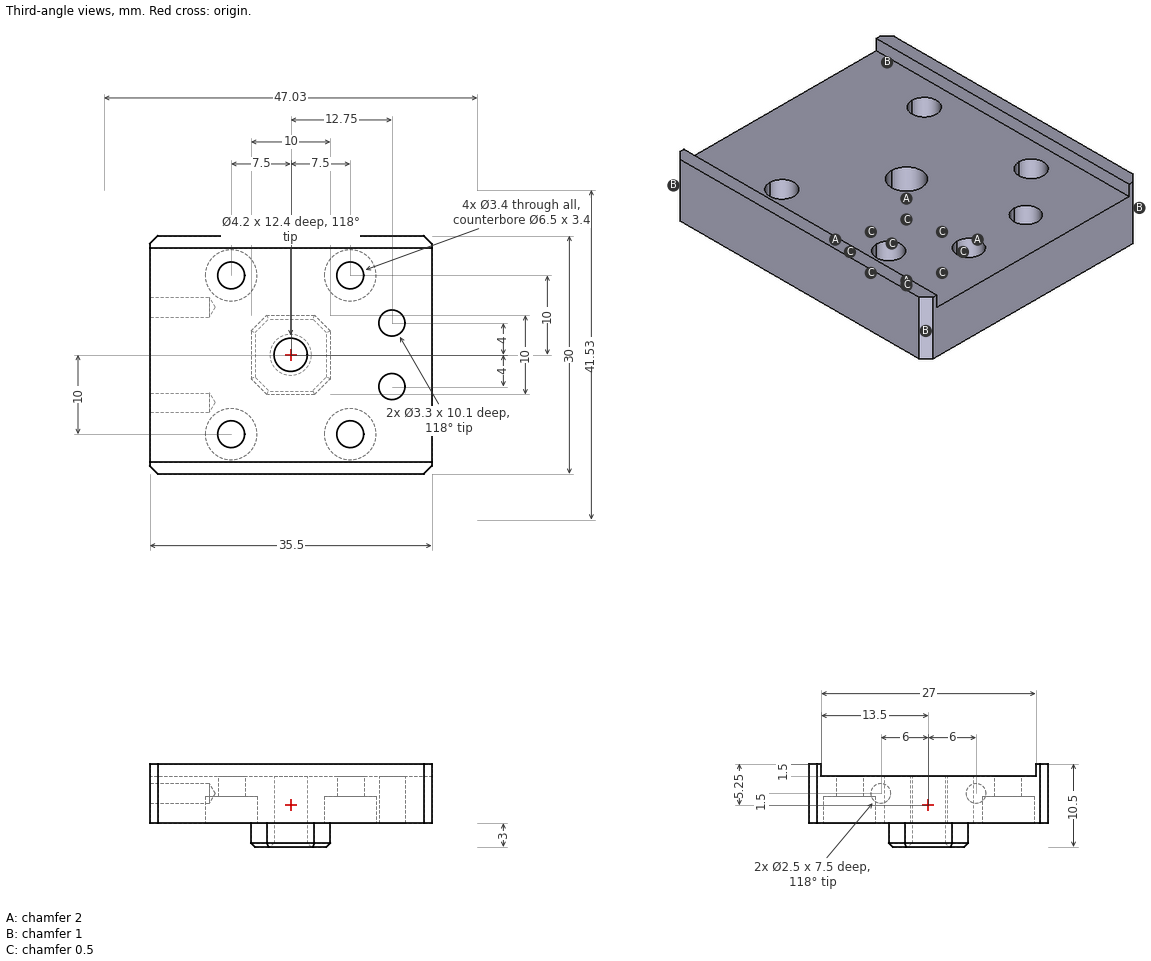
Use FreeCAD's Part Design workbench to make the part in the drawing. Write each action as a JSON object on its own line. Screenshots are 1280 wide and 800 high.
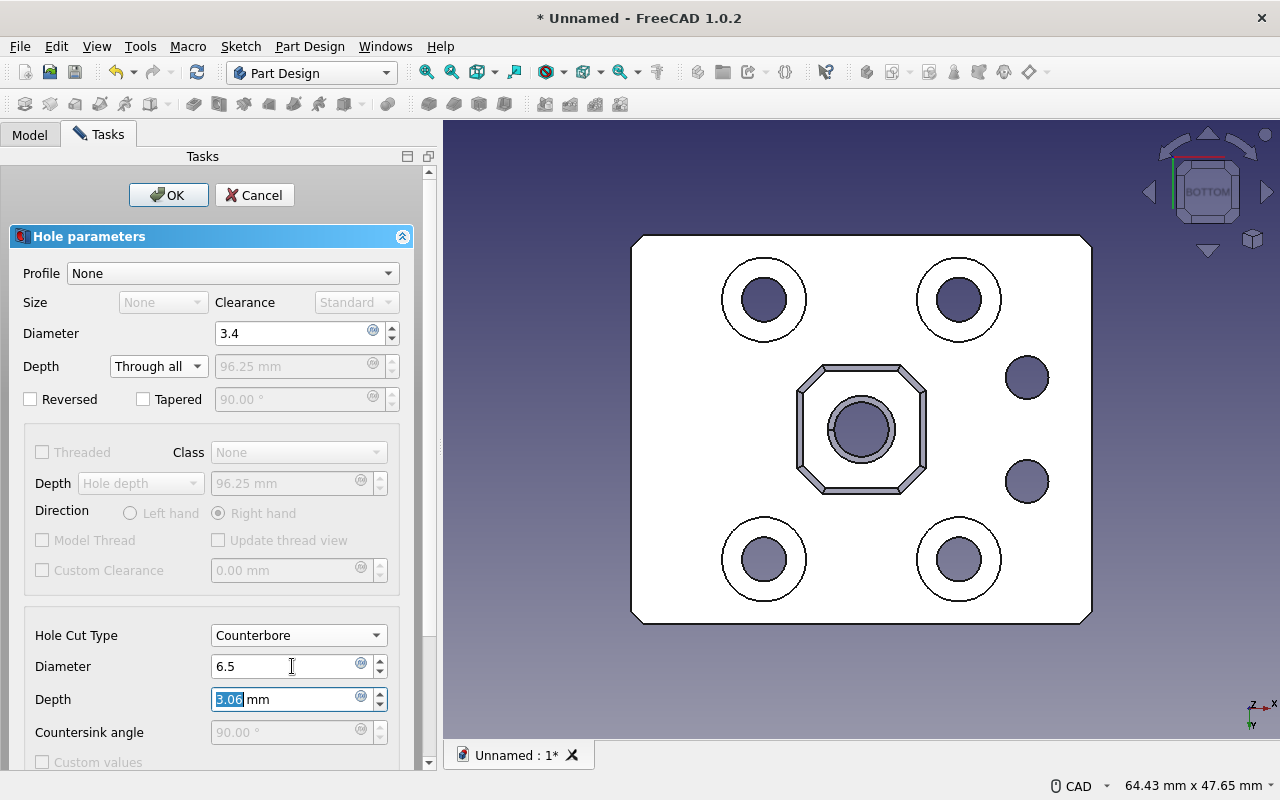
{"action": "type", "text": "3.4"}
{"action": "key", "text": "Tab"}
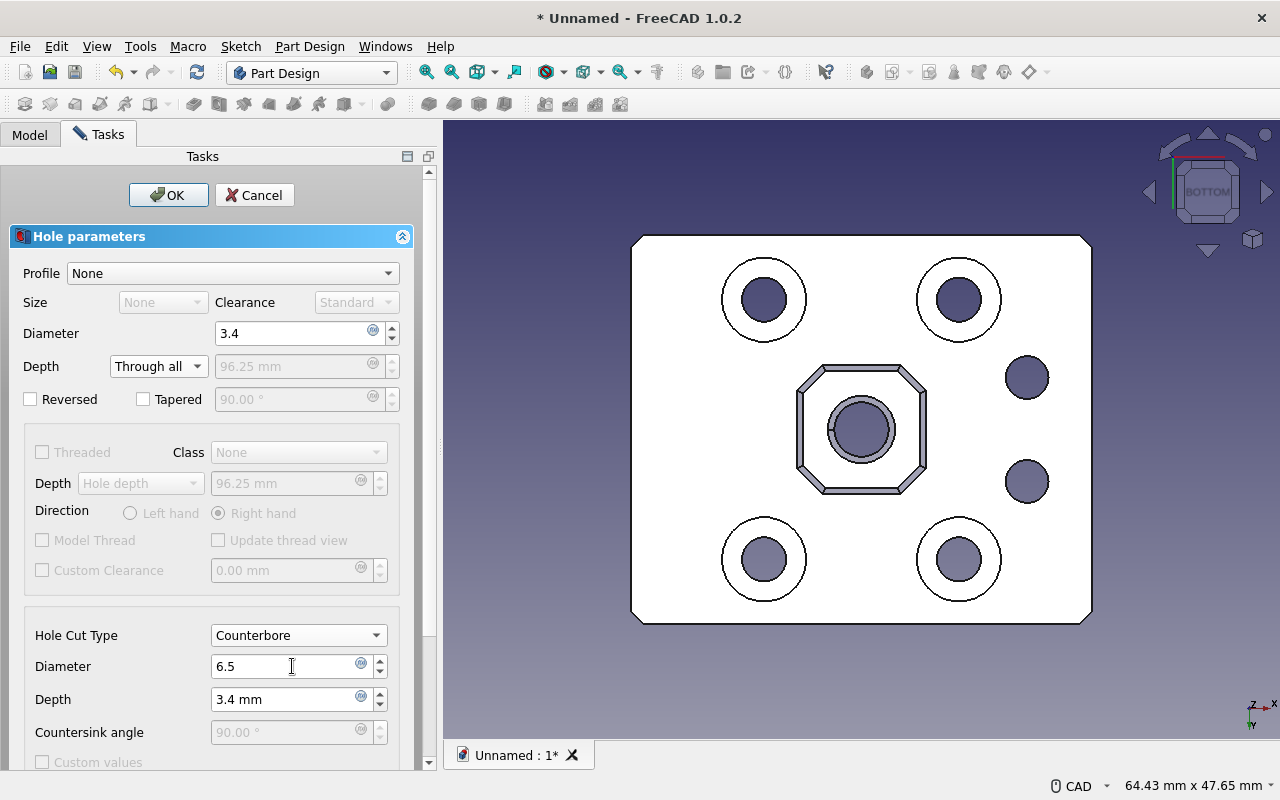
{"action": "left_click", "coordinate": [169, 195]}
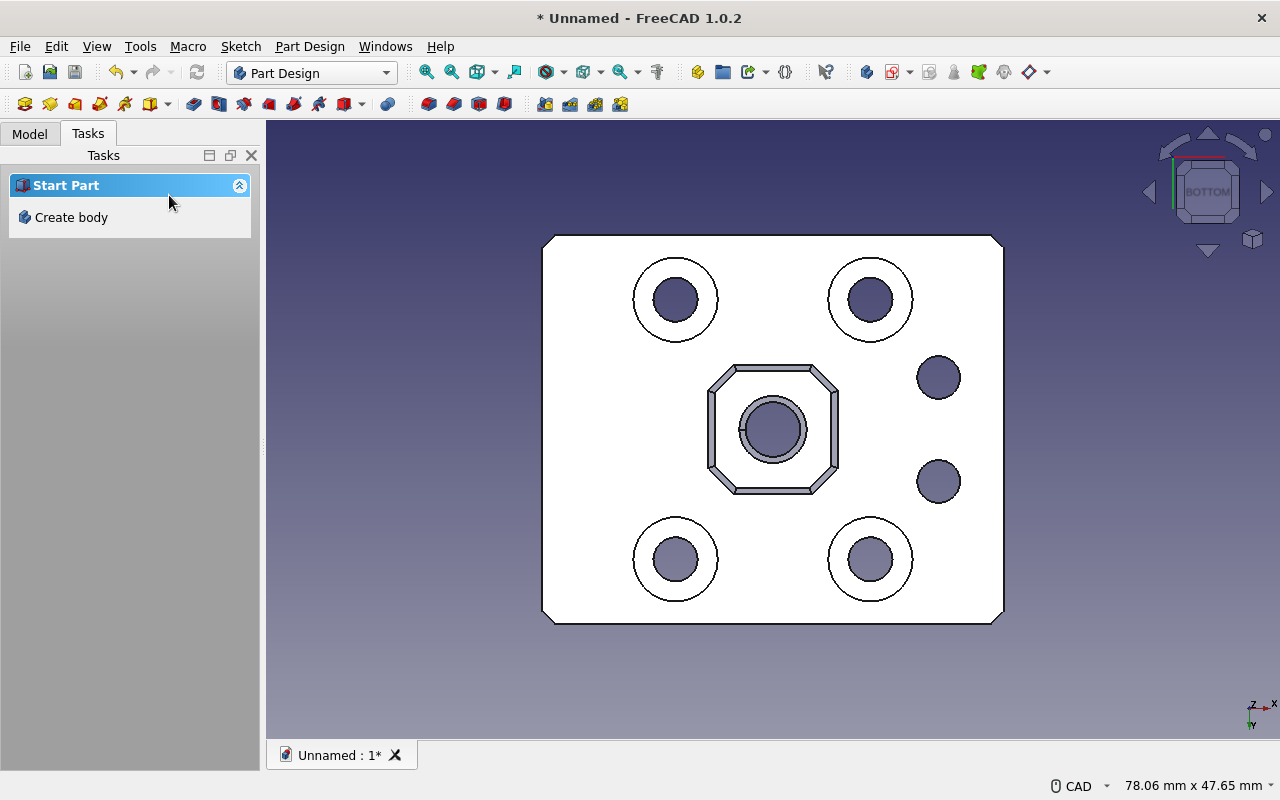
{"action": "key", "text": "6"}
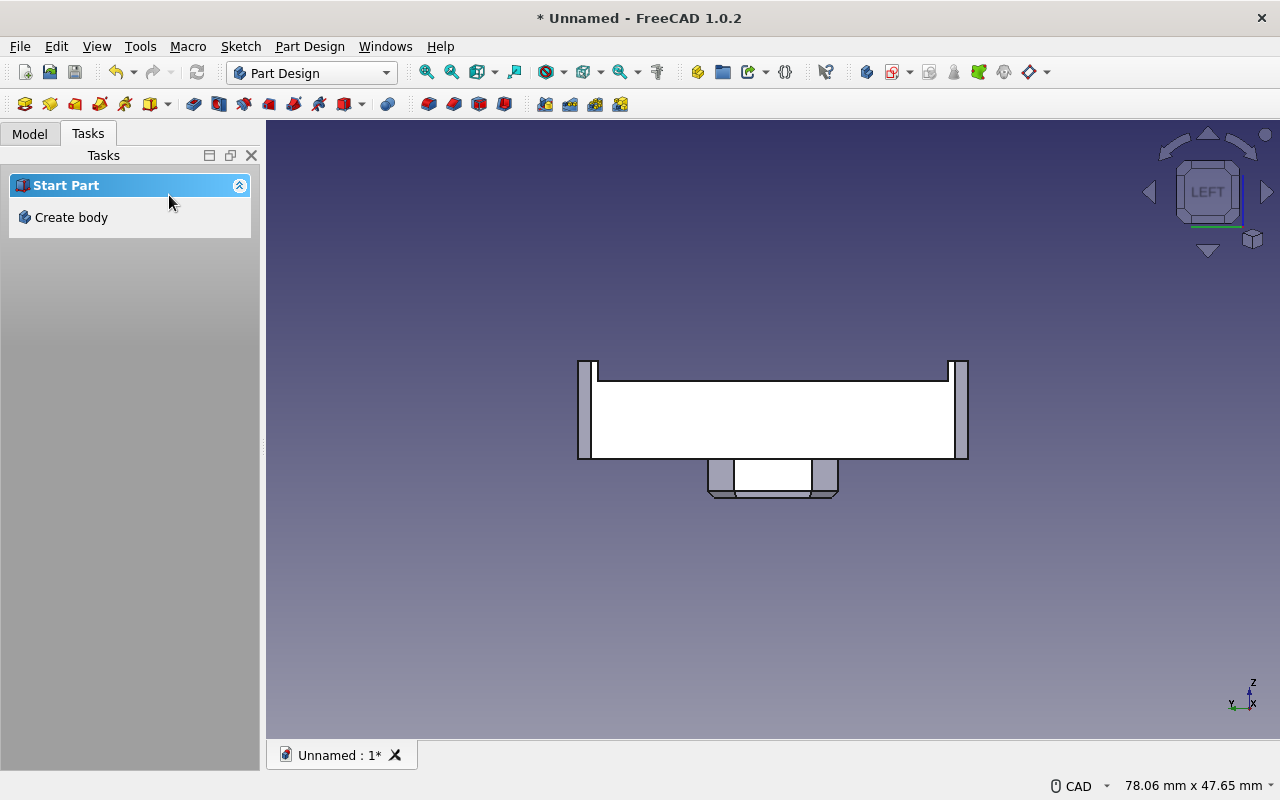
{"action": "left_click", "coordinate": [427, 72]}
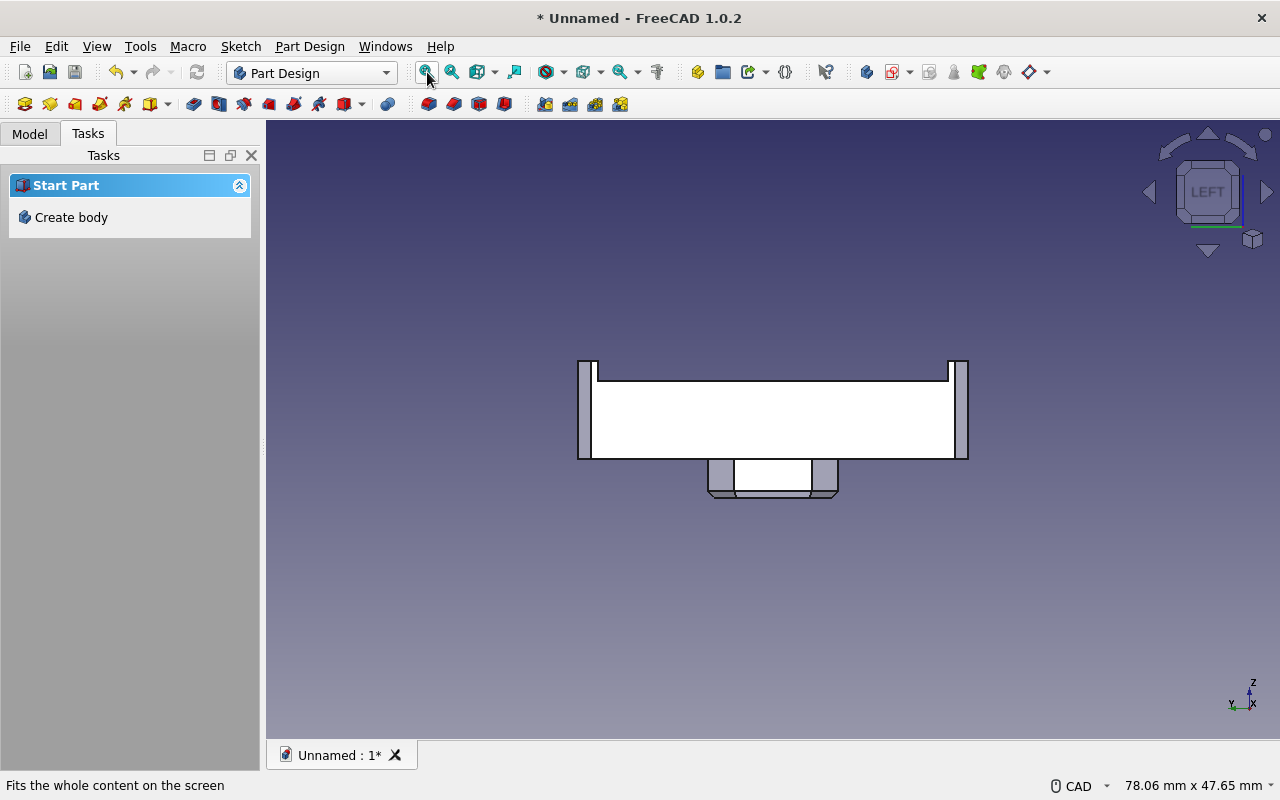
{"action": "left_click", "coordinate": [669, 423]}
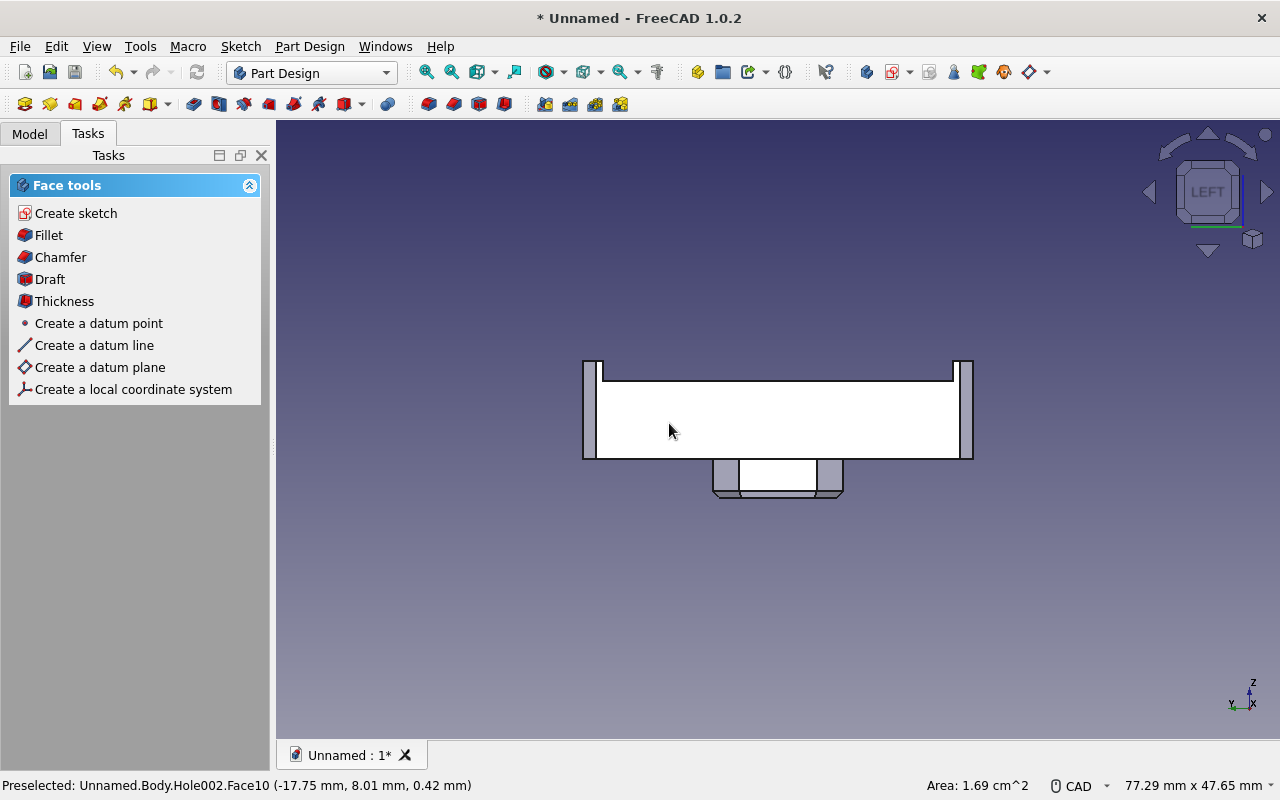
{"action": "left_click", "coordinate": [892, 72]}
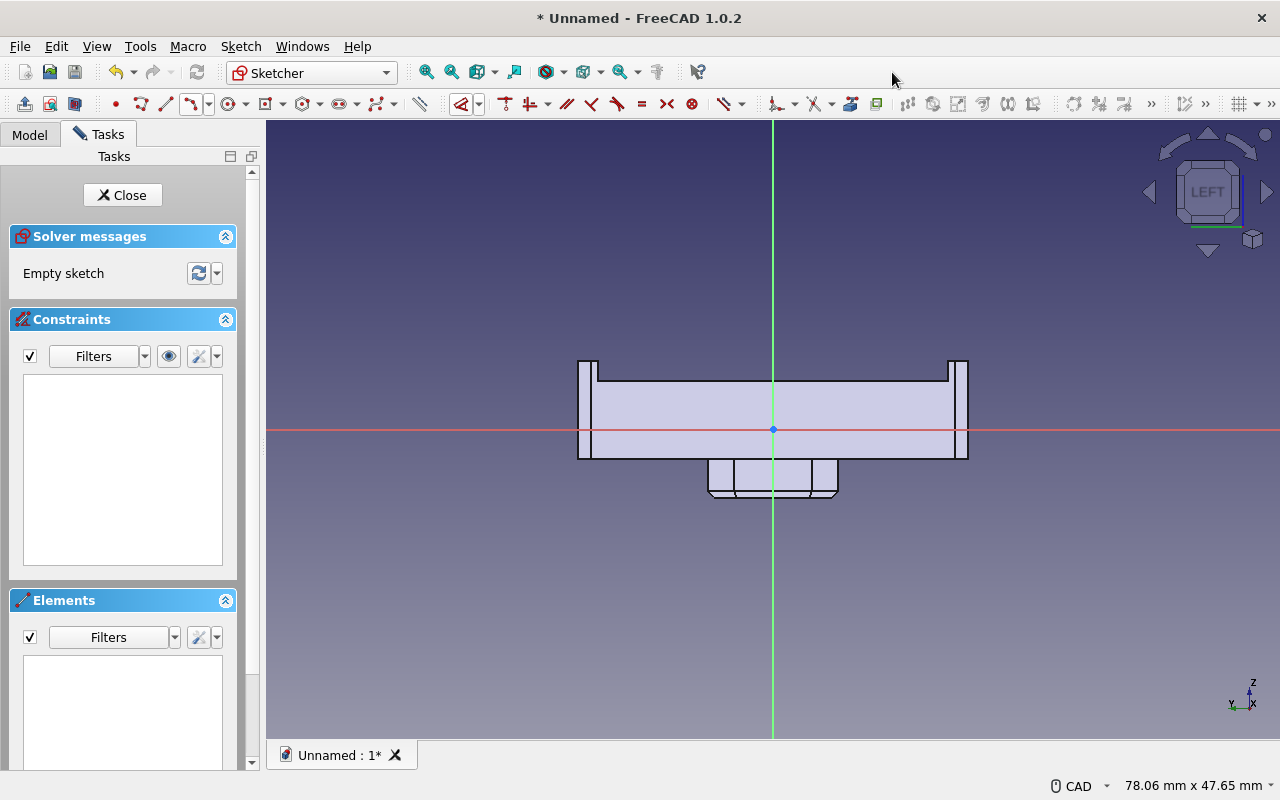
{"action": "scroll", "coordinate": [803, 404], "scroll_direction": "up", "scroll_amount": 6}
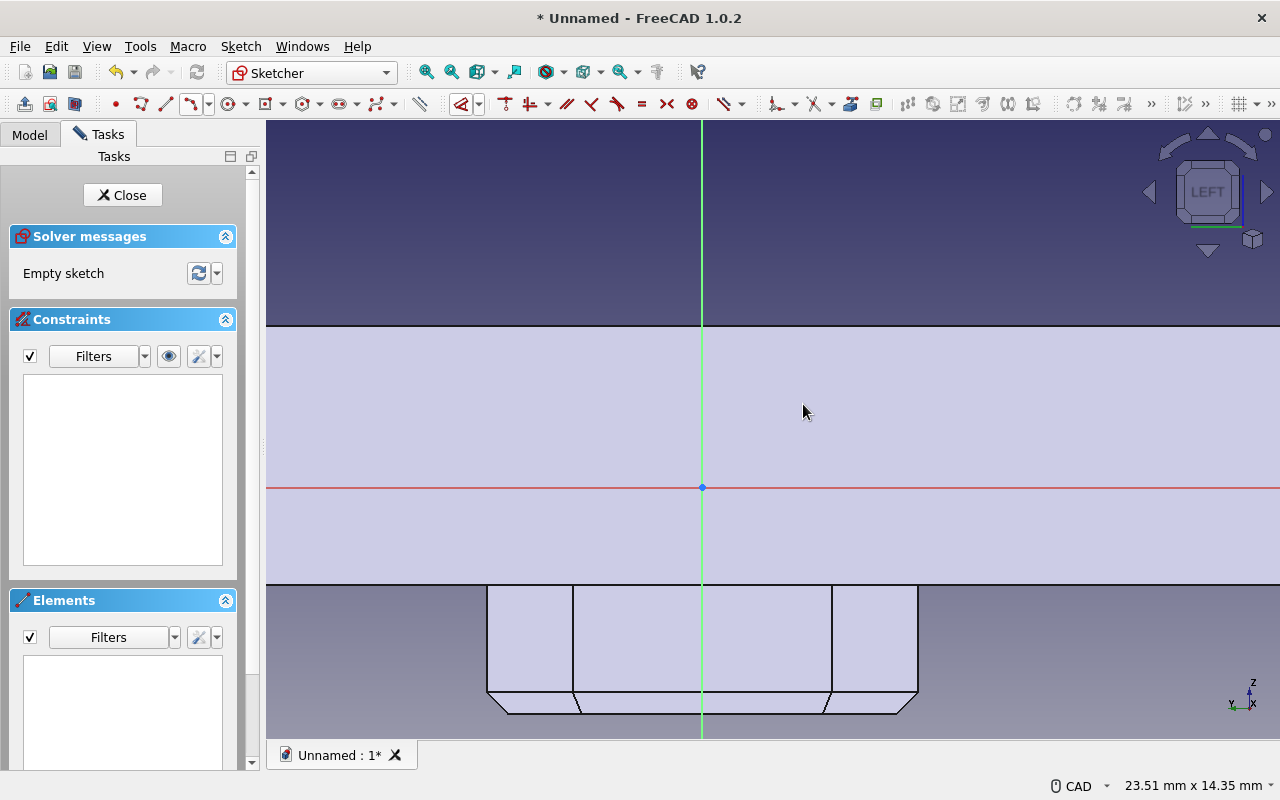
{"action": "key", "text": "g c"}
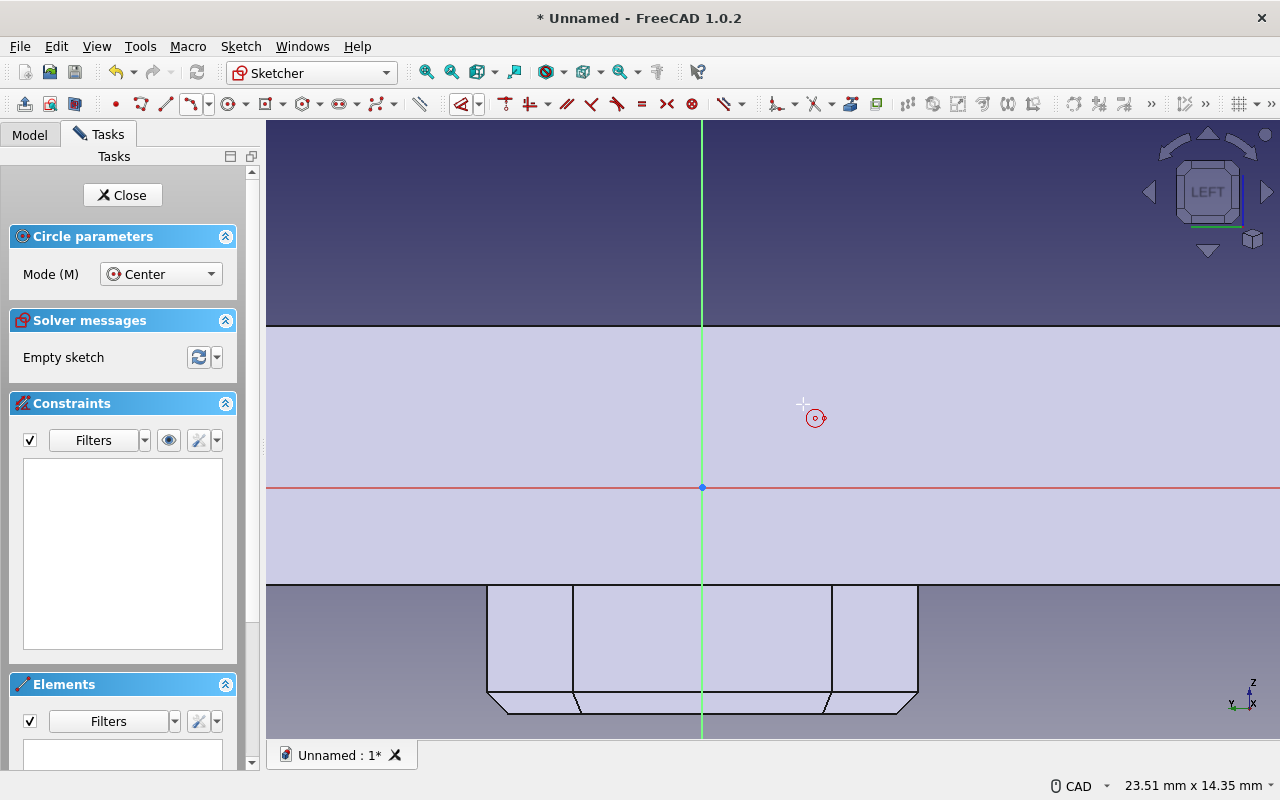
{"action": "left_click", "coordinate": [961, 423]}
{"action": "left_click", "coordinate": [999, 385]}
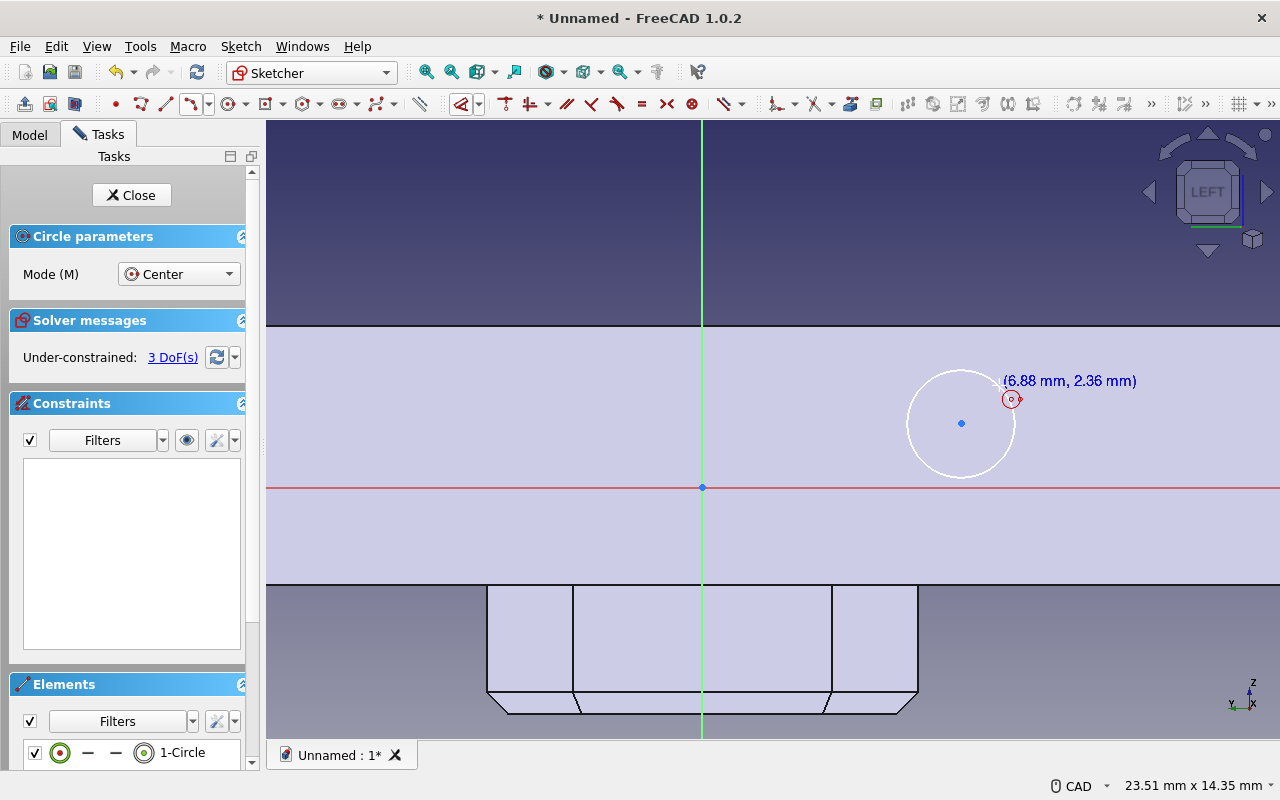
{"action": "left_click", "coordinate": [443, 423]}
{"action": "left_click", "coordinate": [482, 385]}
{"action": "key", "text": "Escape"}